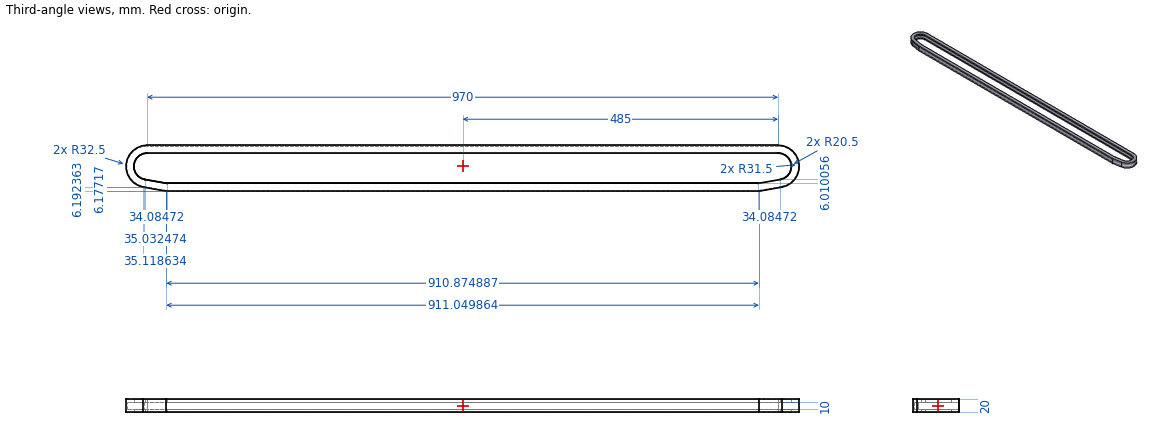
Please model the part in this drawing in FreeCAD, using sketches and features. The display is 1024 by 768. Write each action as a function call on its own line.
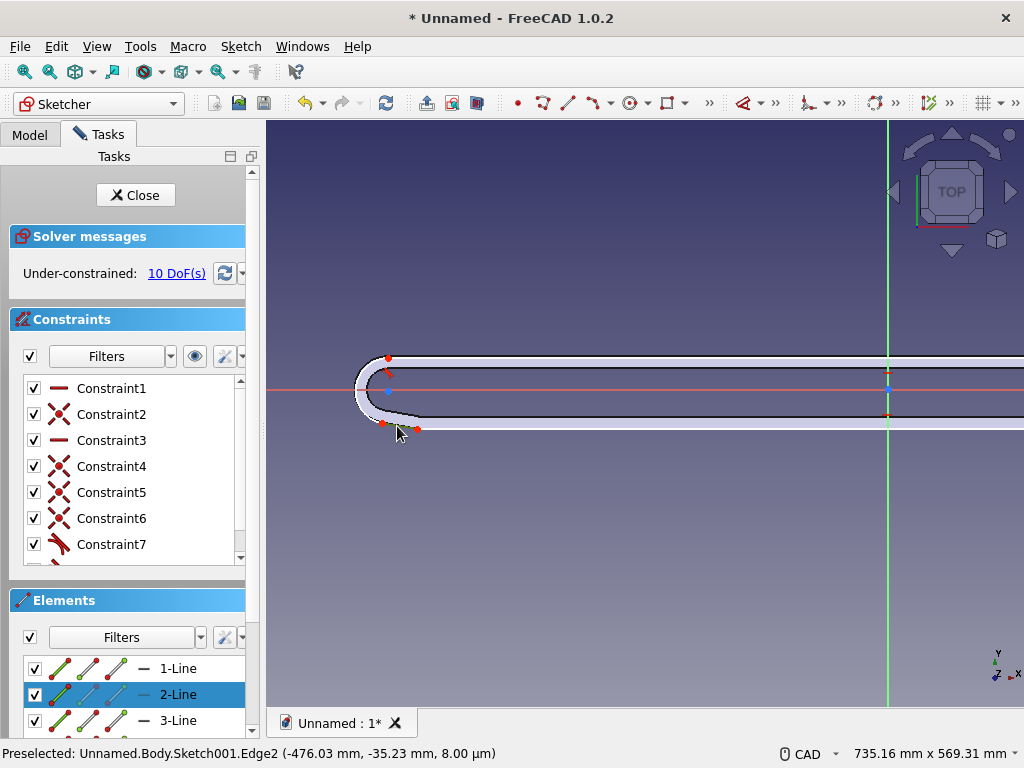
click(363, 370)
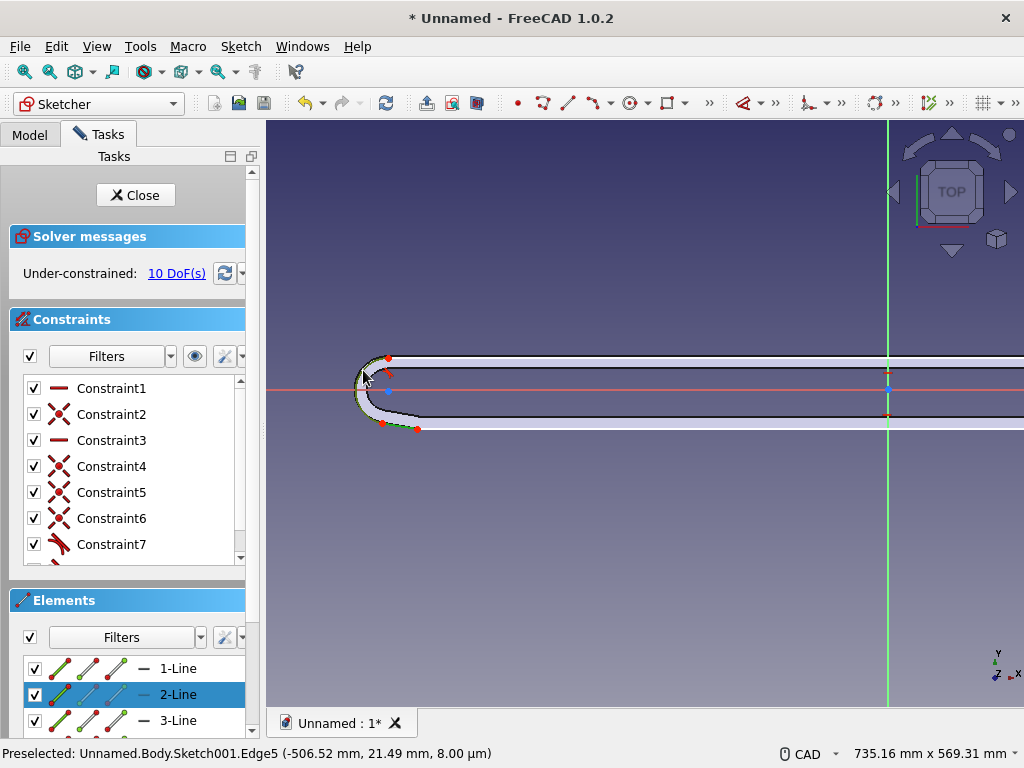
key(t)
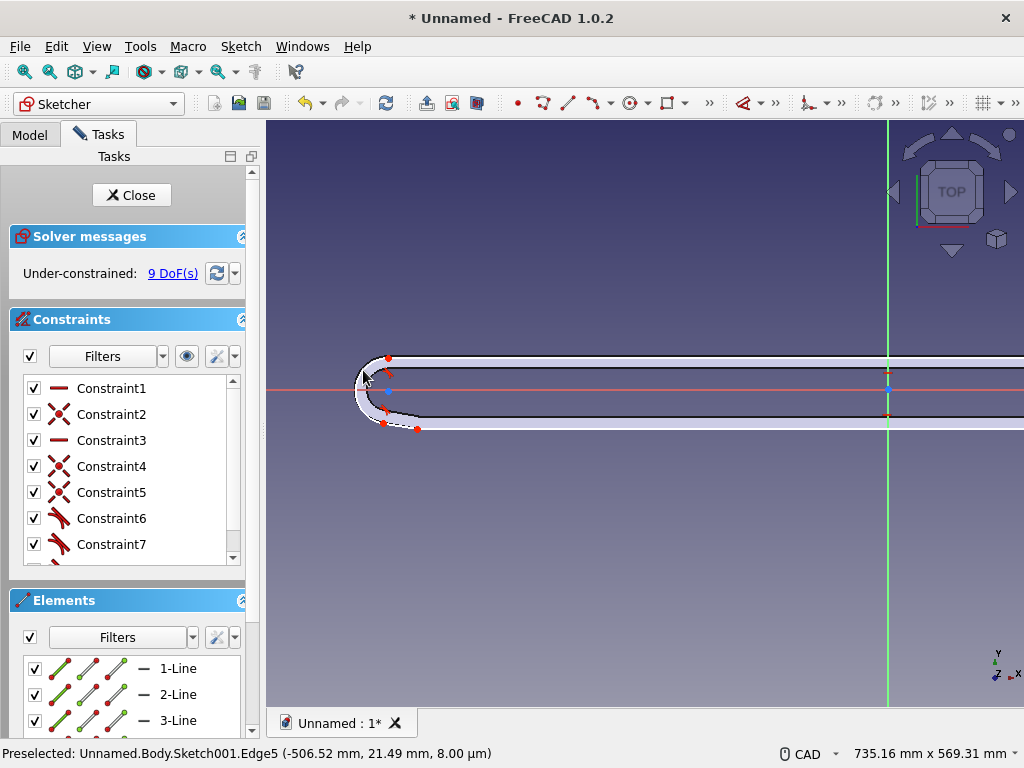
scroll(395, 426, down, 5)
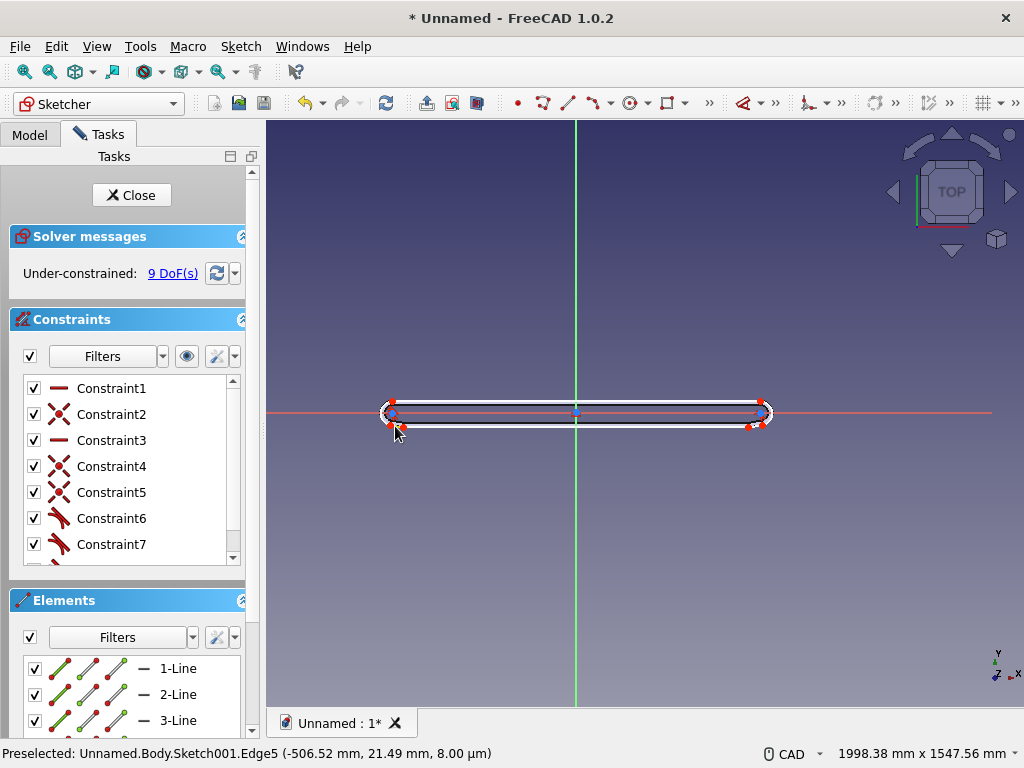
scroll(753, 427, up, 7)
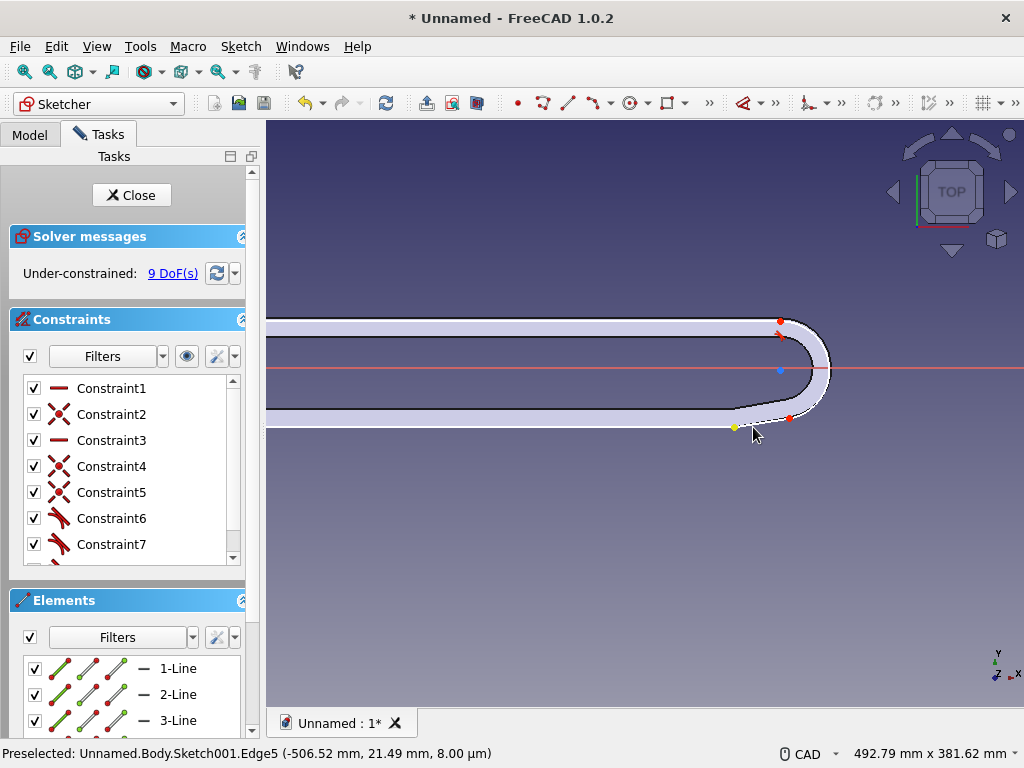
click(751, 425)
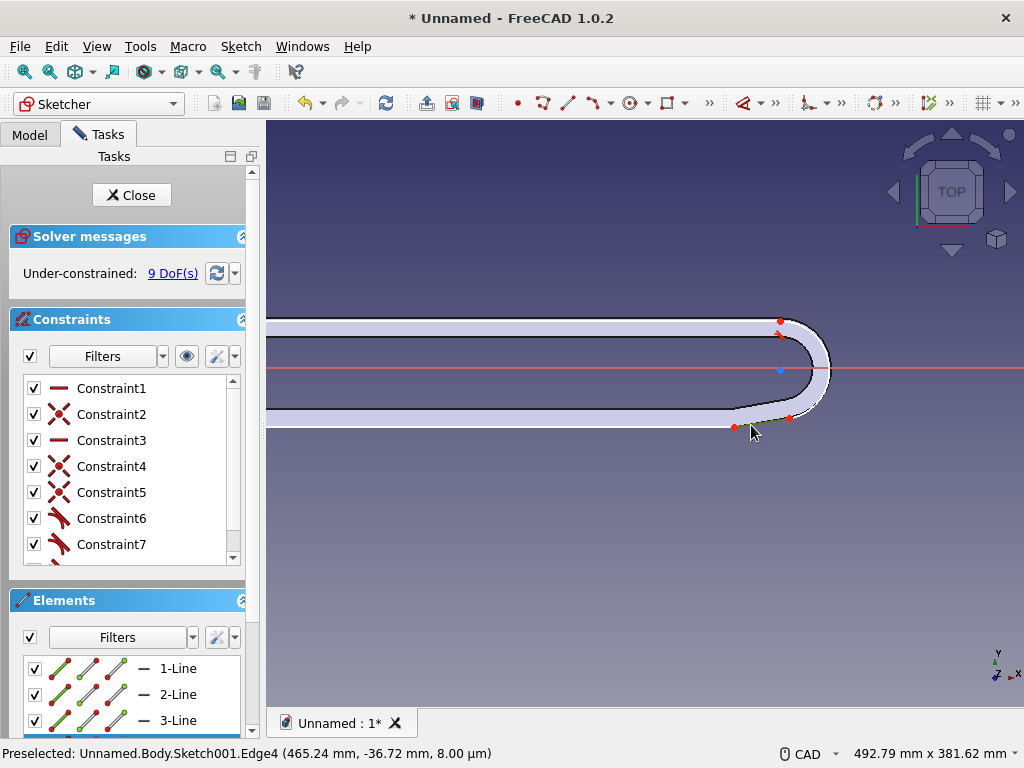
click(823, 394)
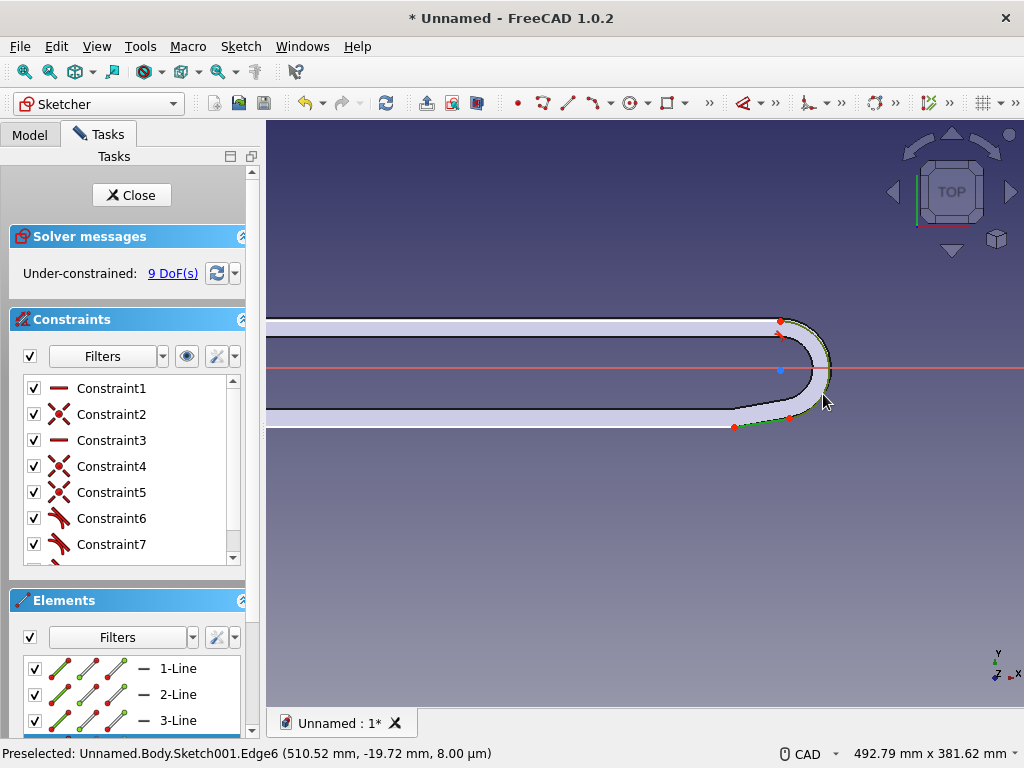
key(t)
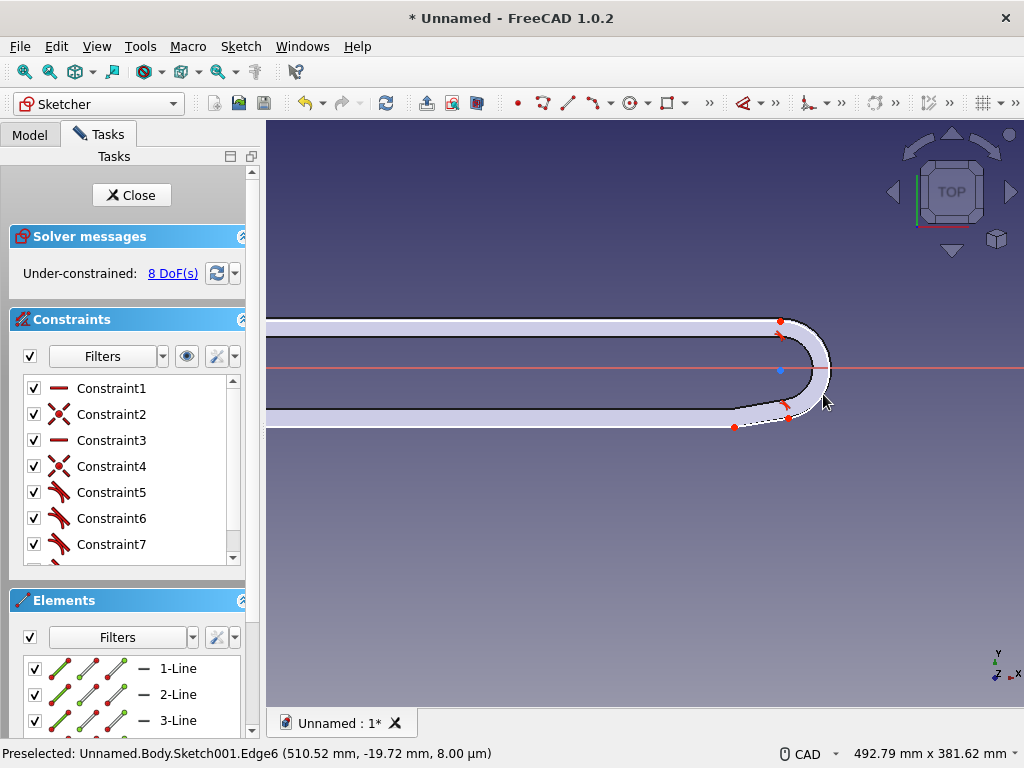
scroll(754, 427, down, 7)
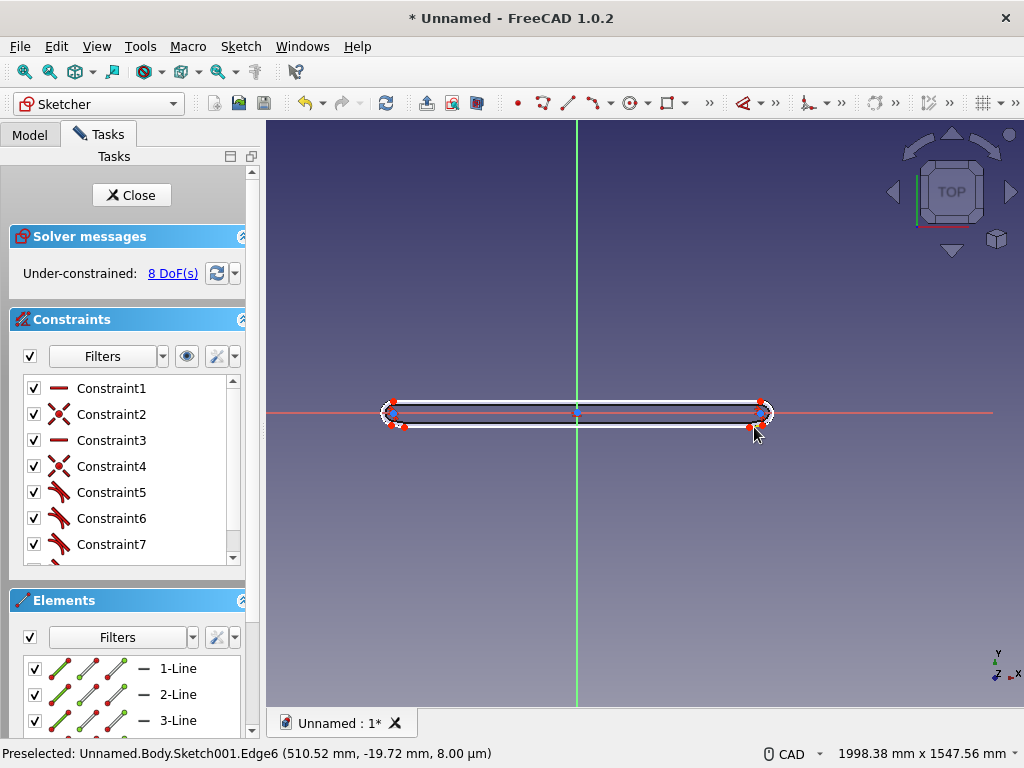
scroll(384, 406, up, 4)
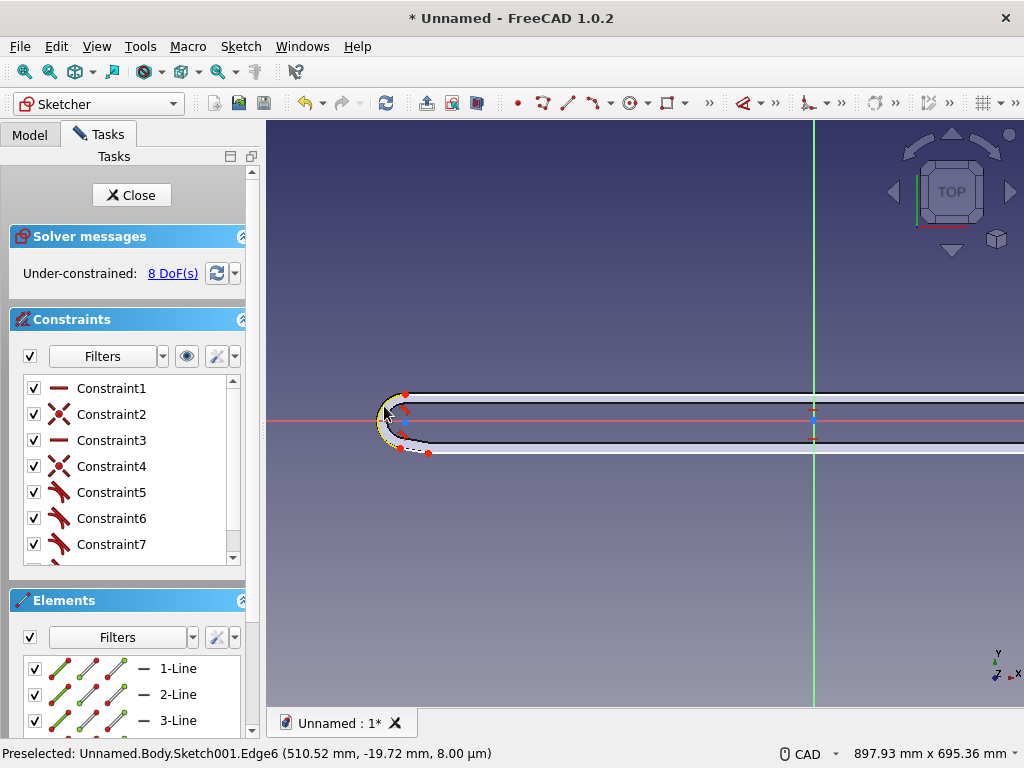
click(384, 405)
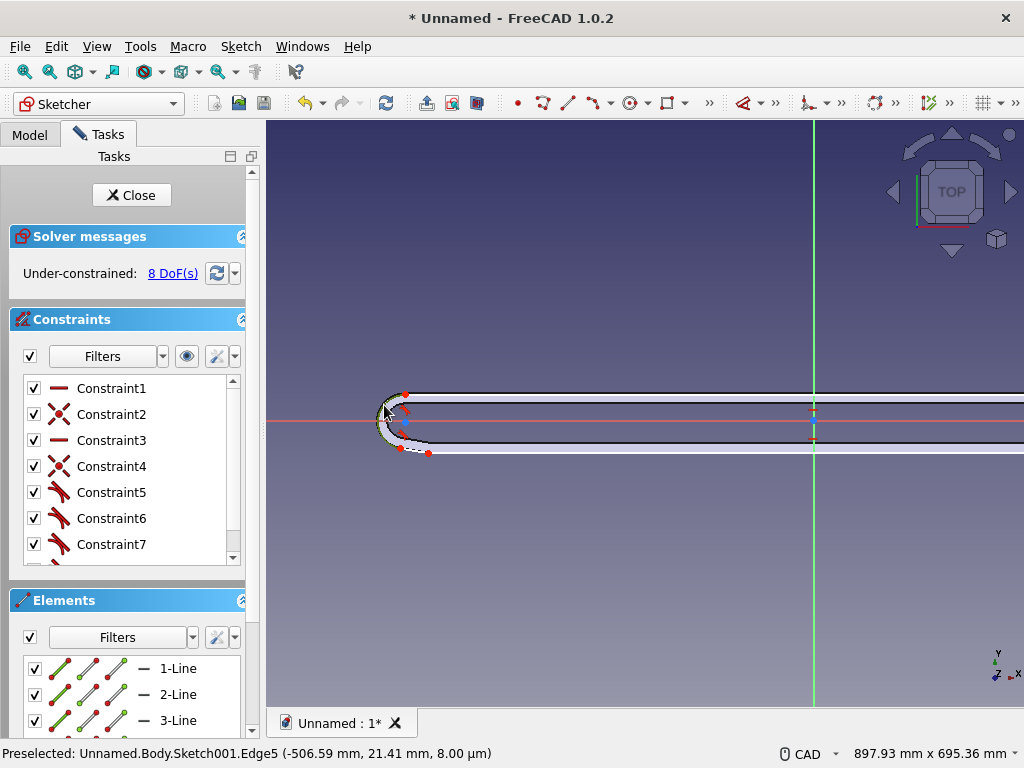
scroll(383, 406, down, 4)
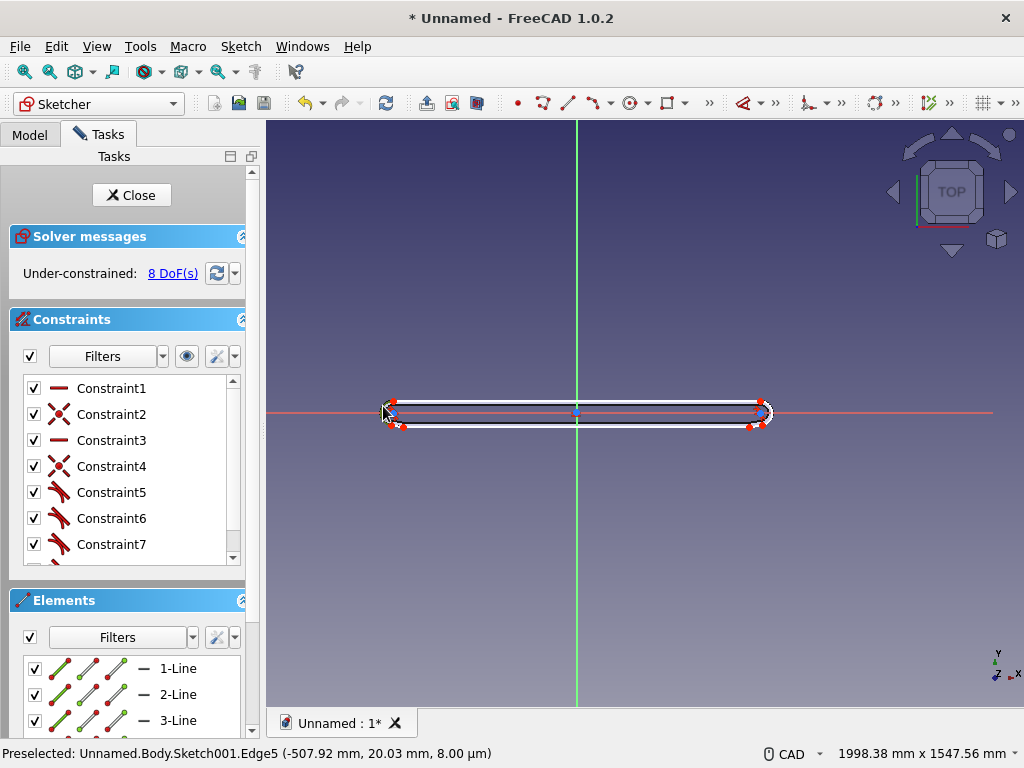
scroll(771, 419, up, 4)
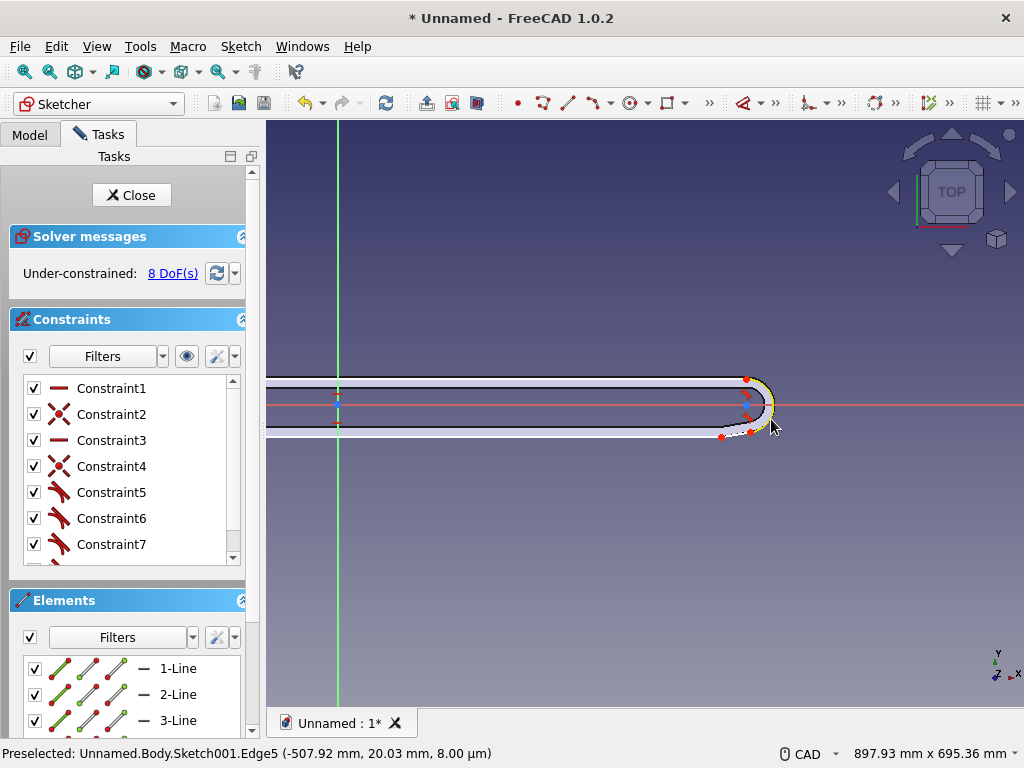
click(770, 419)